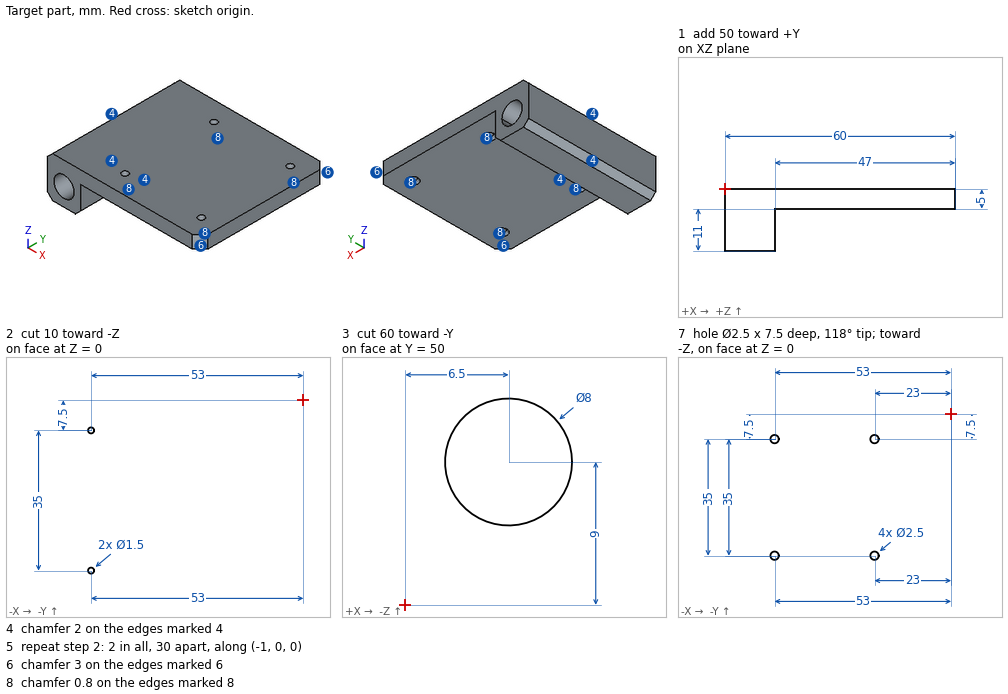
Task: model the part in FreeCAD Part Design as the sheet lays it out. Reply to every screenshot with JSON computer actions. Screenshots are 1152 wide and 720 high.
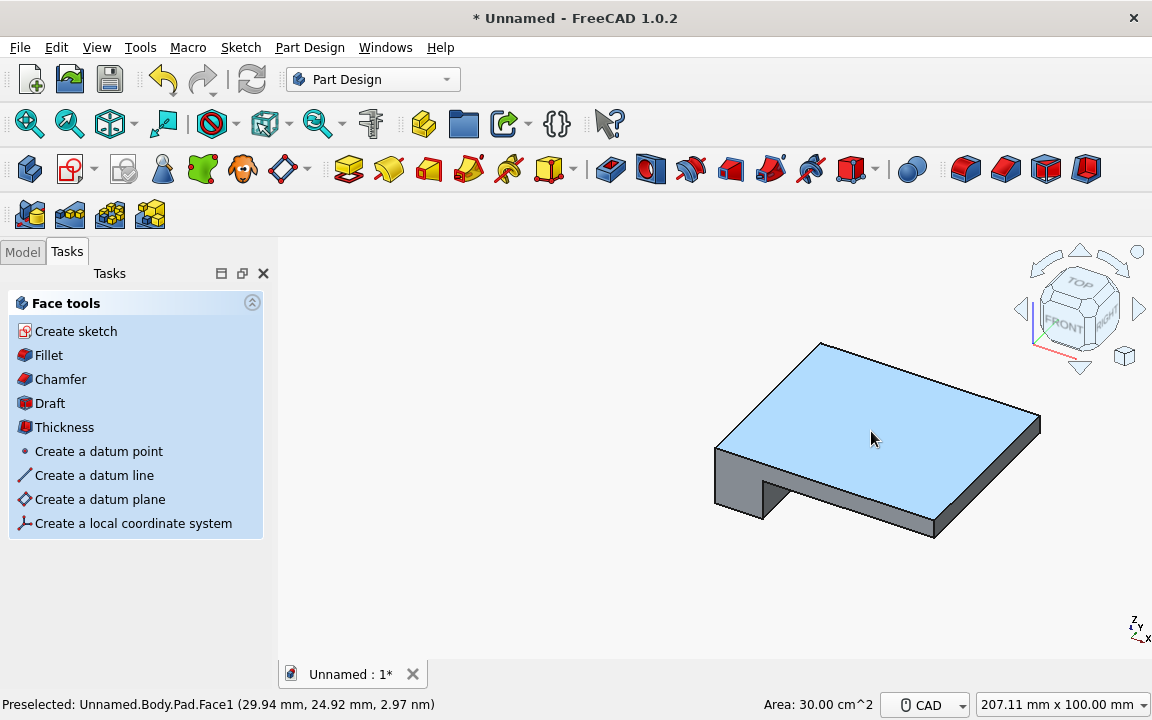
{"action": "left_click", "coordinate": [70, 170]}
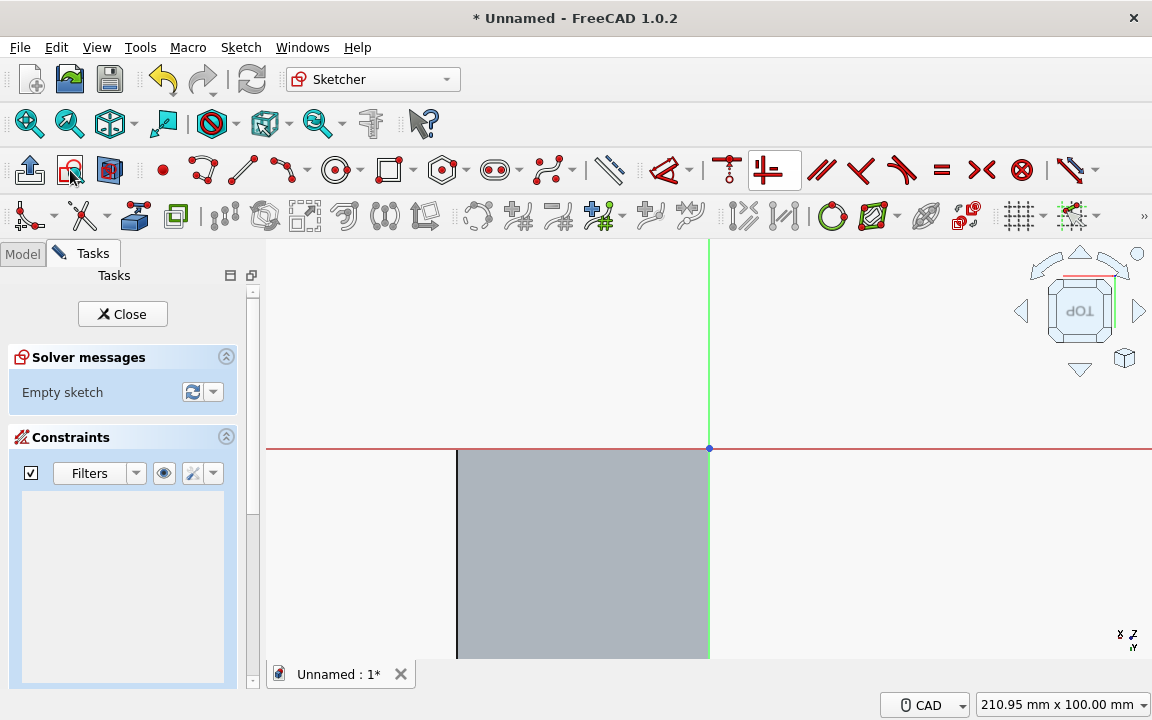
{"action": "scroll", "coordinate": [841, 267], "scroll_direction": "down", "scroll_amount": 1}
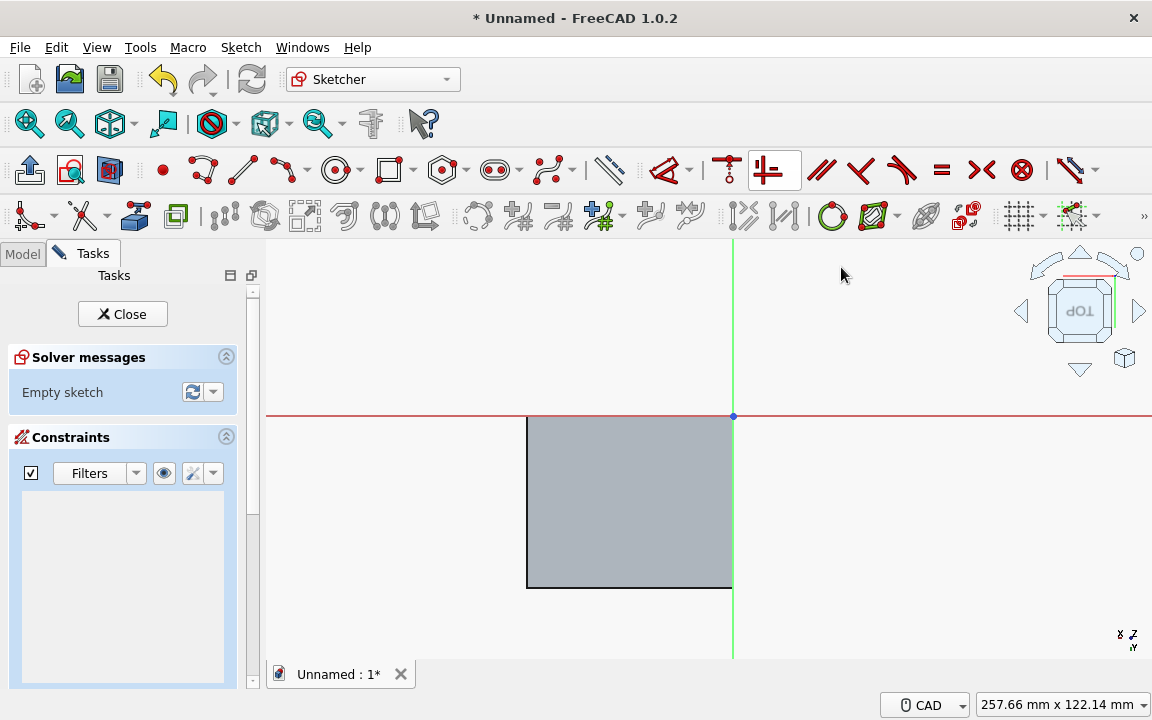
{"action": "scroll", "coordinate": [641, 541], "scroll_direction": "up", "scroll_amount": 3}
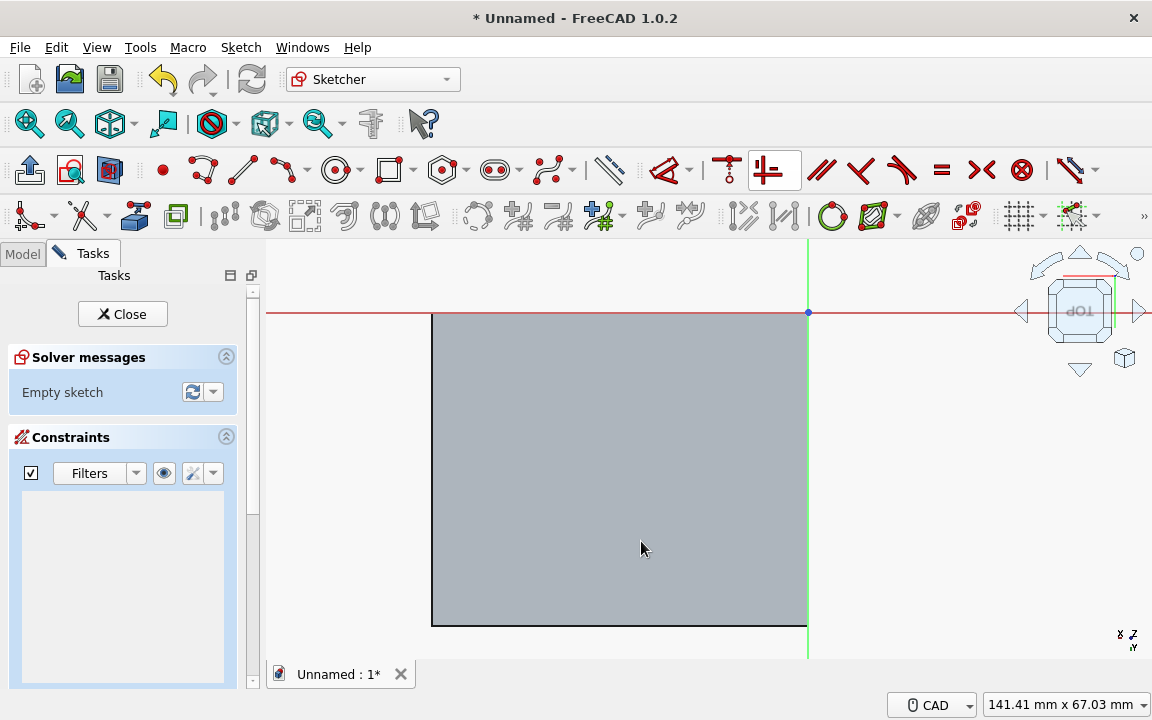
{"action": "left_click", "coordinate": [336, 170]}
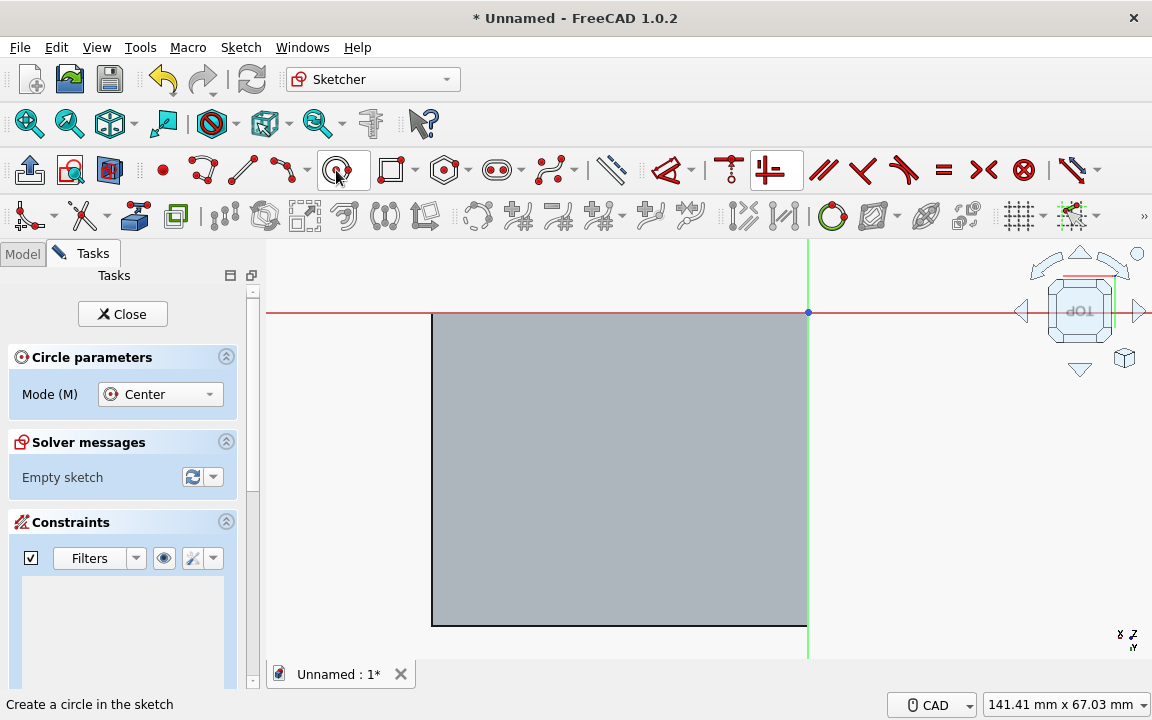
{"action": "scroll", "coordinate": [476, 579], "scroll_direction": "up", "scroll_amount": 8}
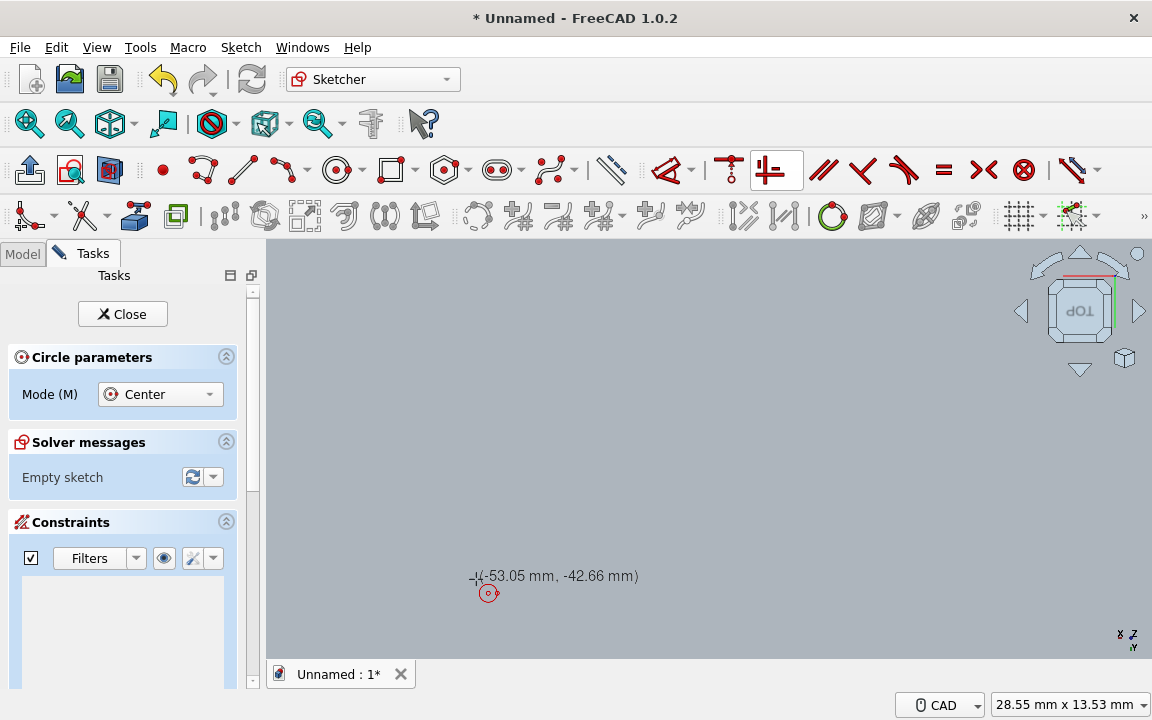
{"action": "scroll", "coordinate": [477, 581], "scroll_direction": "down", "scroll_amount": 8}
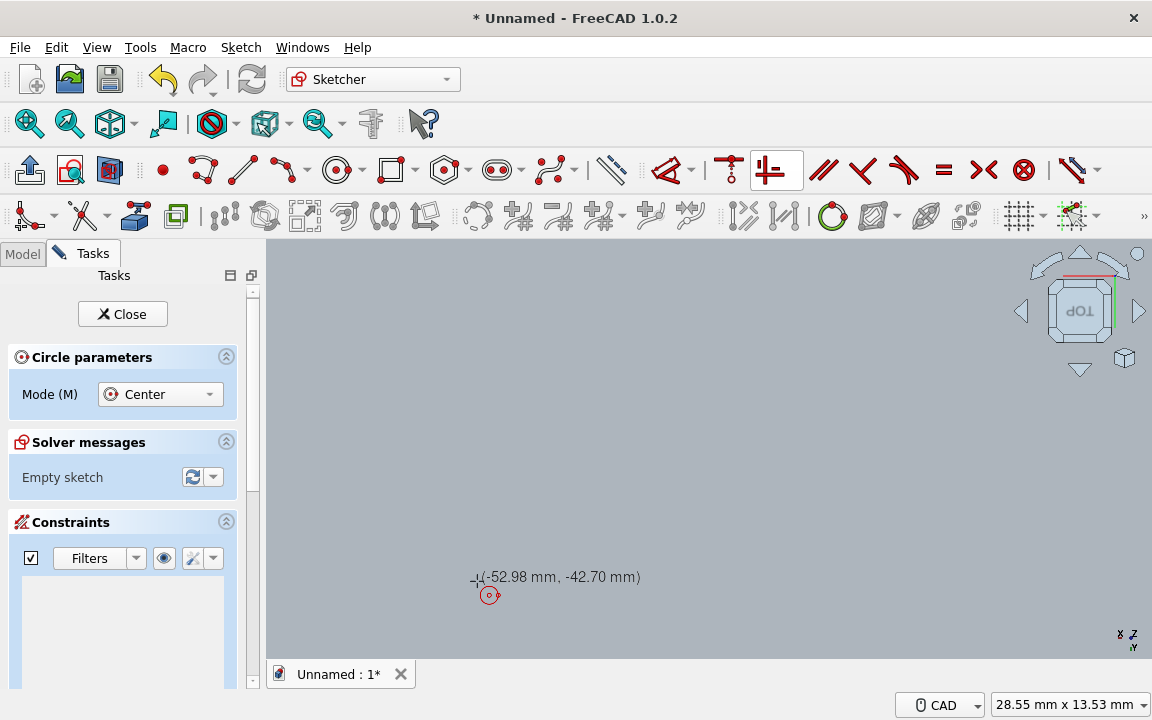
{"action": "left_click", "coordinate": [477, 581]}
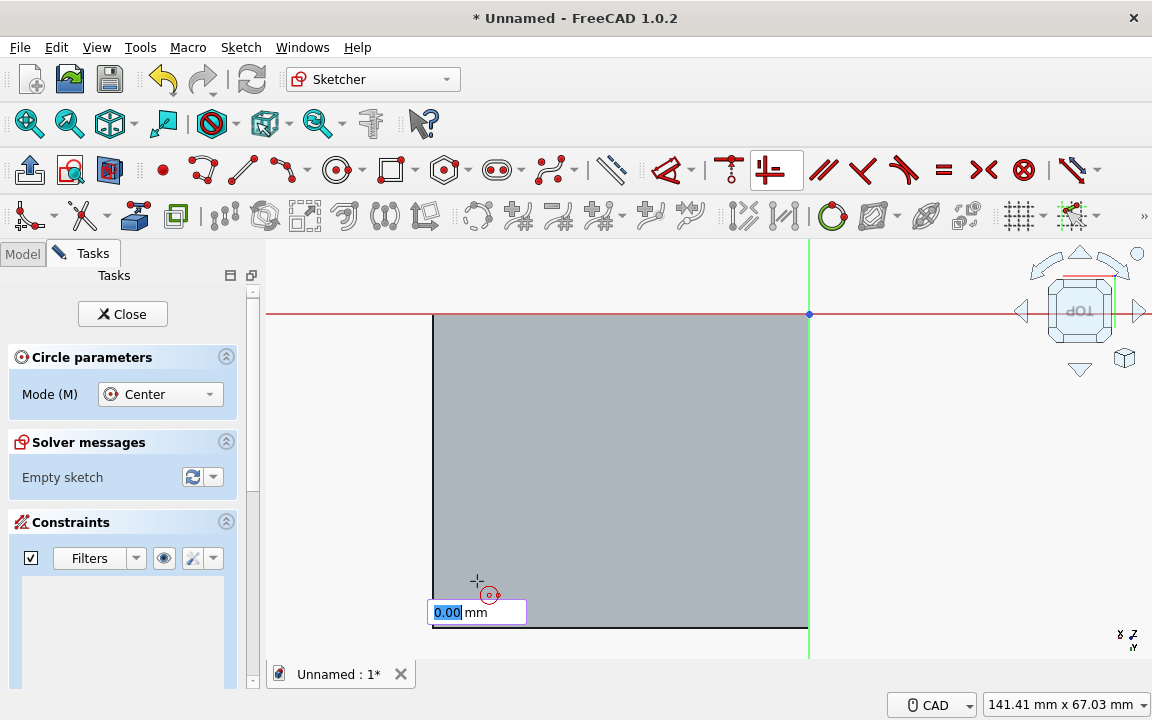
{"action": "scroll", "coordinate": [480, 577], "scroll_direction": "up", "scroll_amount": 7}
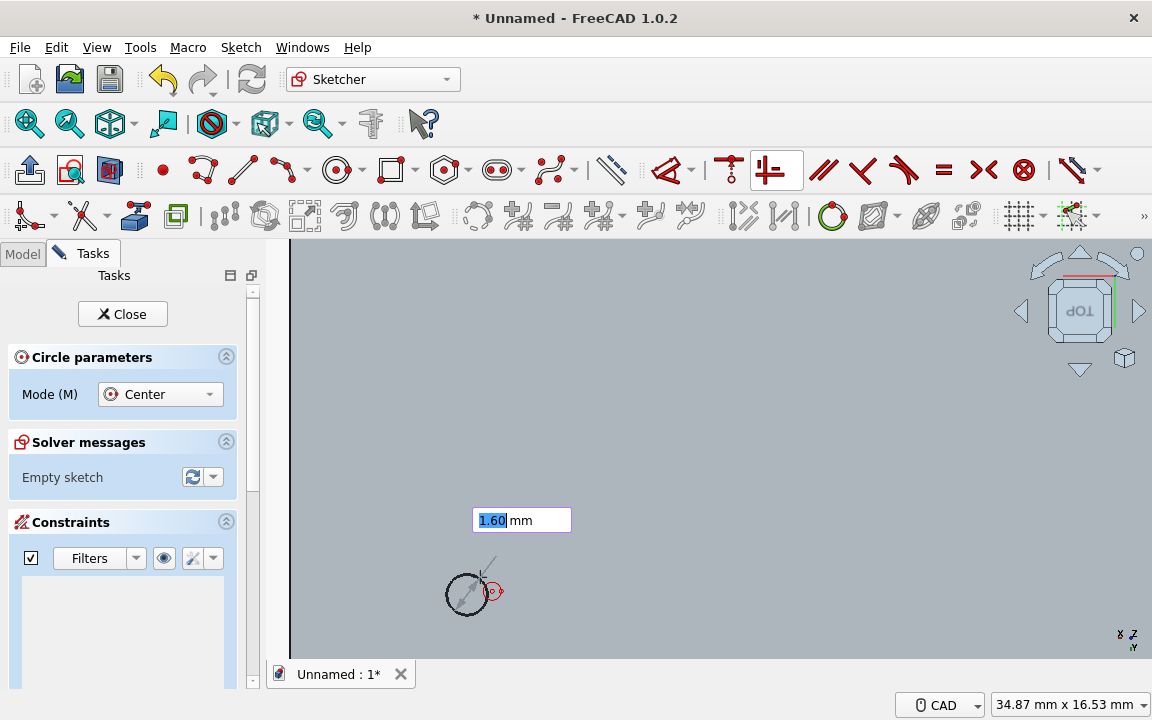
{"action": "left_click", "coordinate": [481, 576]}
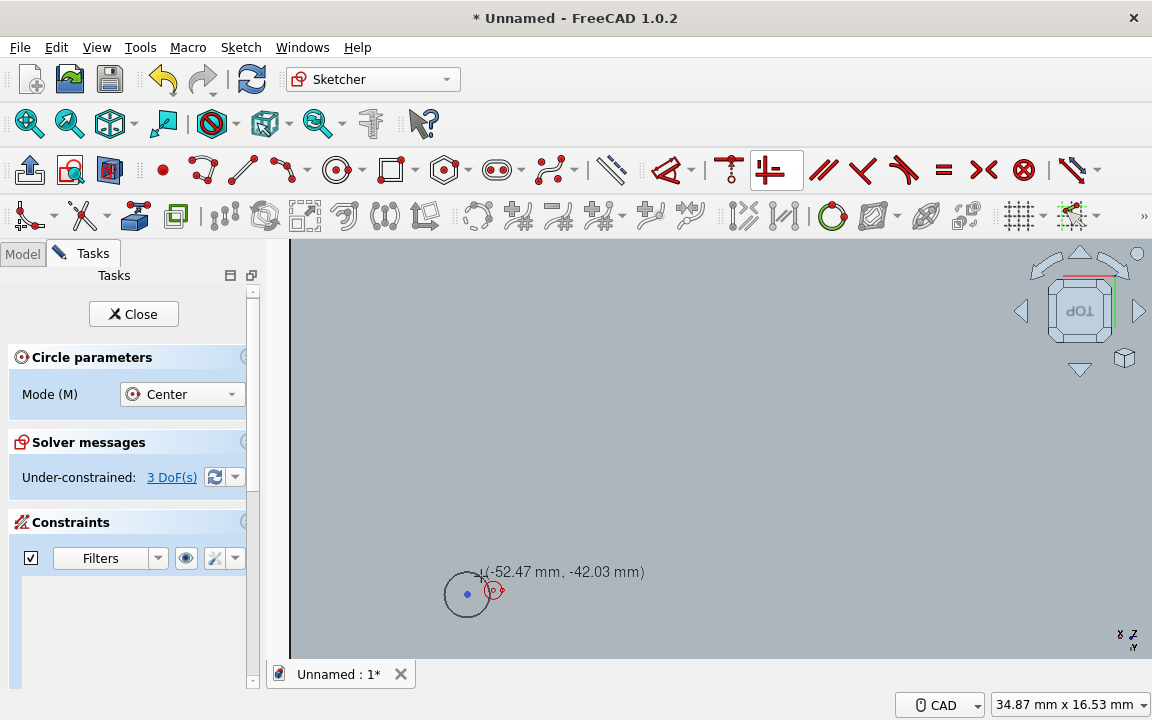
{"action": "scroll", "coordinate": [480, 577], "scroll_direction": "down", "scroll_amount": 7}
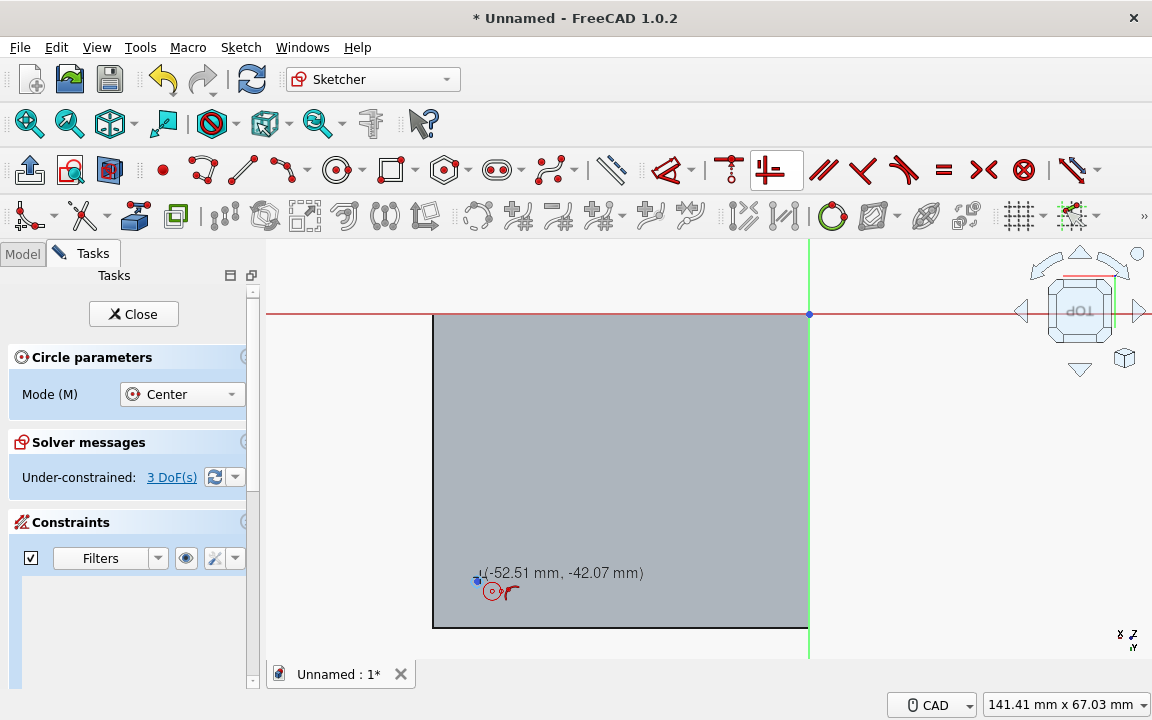
{"action": "scroll", "coordinate": [477, 361], "scroll_direction": "up", "scroll_amount": 8}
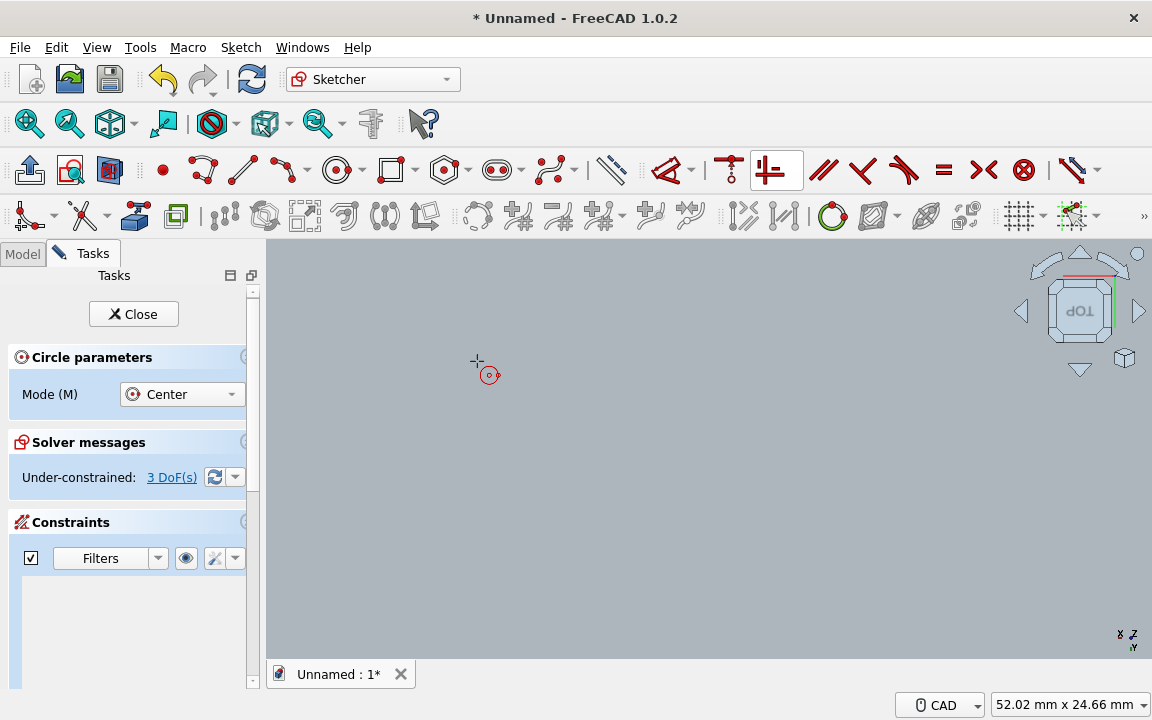
{"action": "scroll", "coordinate": [477, 360], "scroll_direction": "down", "scroll_amount": 8}